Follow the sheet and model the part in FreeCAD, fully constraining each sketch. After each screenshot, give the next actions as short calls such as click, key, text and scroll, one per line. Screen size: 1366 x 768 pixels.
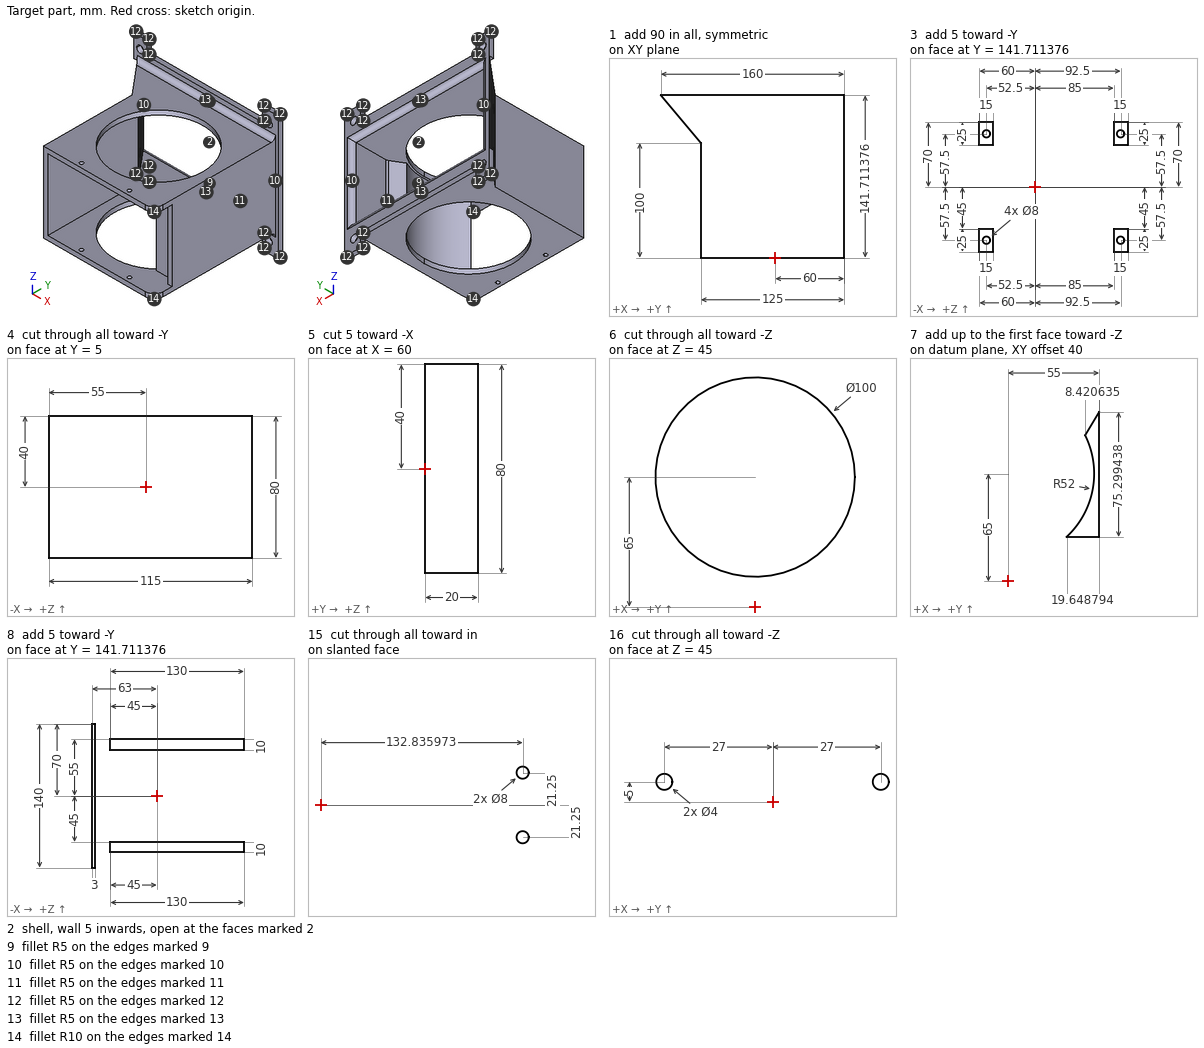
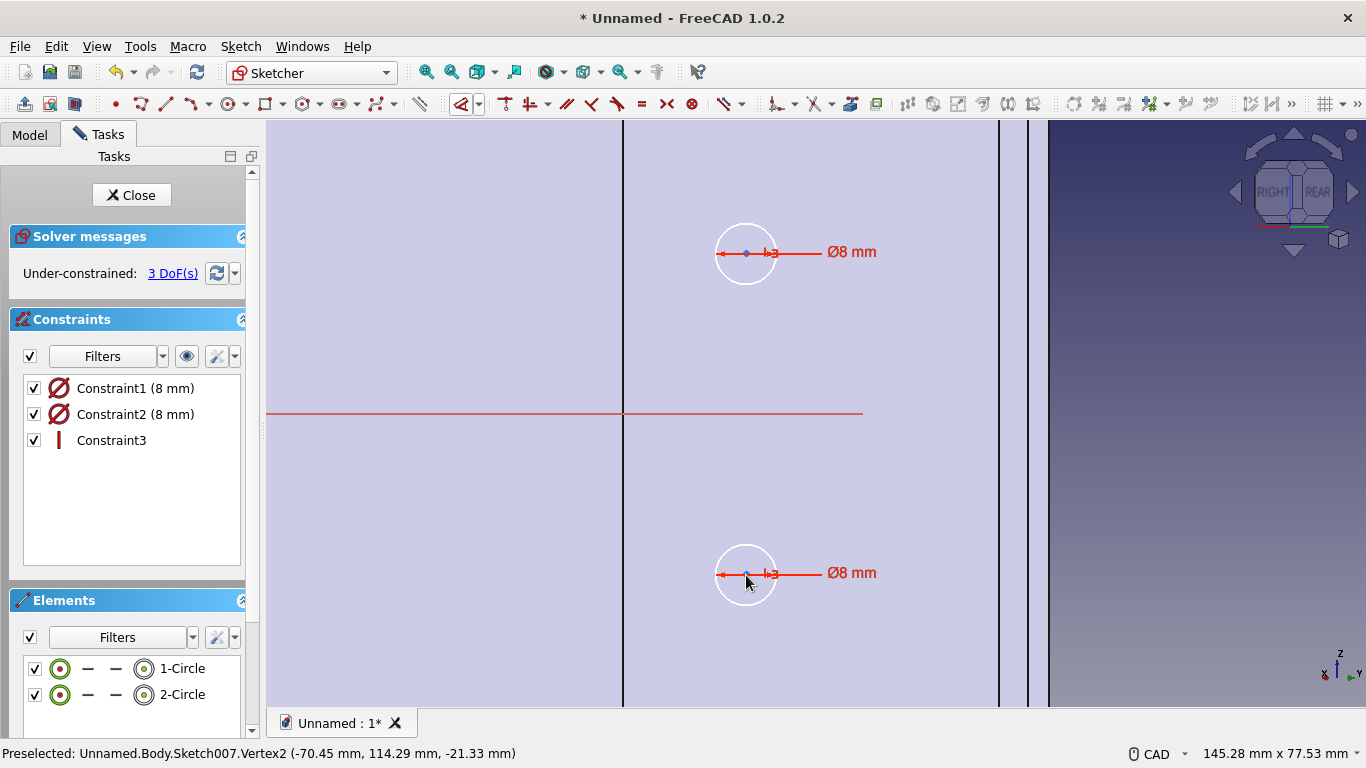
click(746, 254)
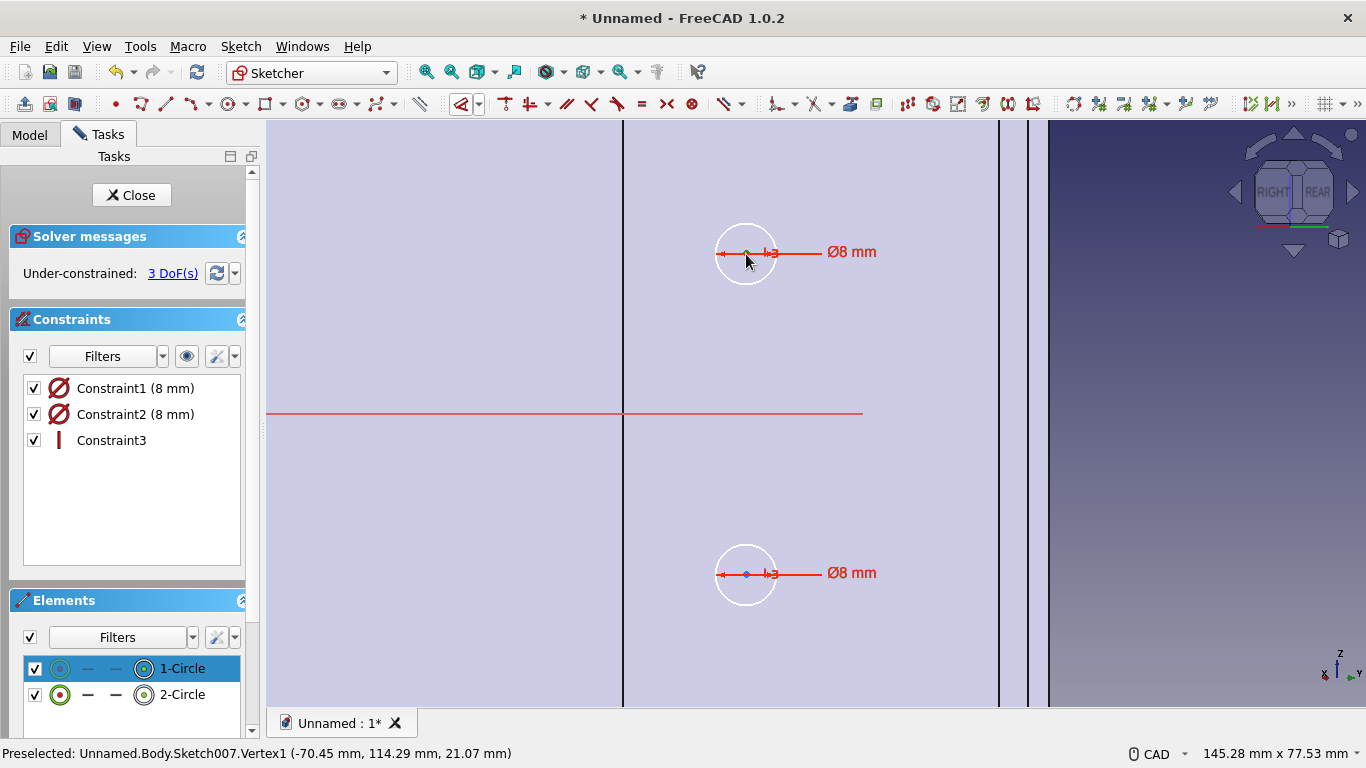
click(478, 104)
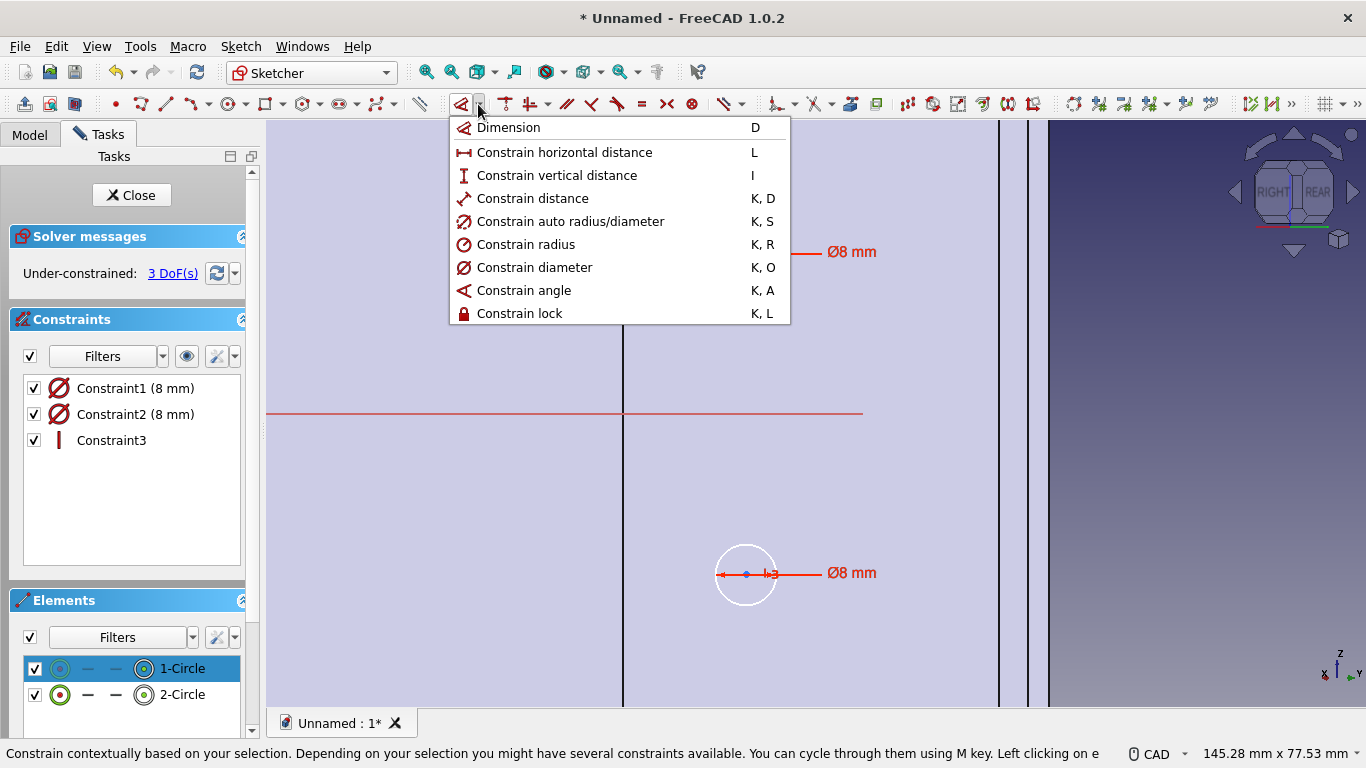
click(620, 176)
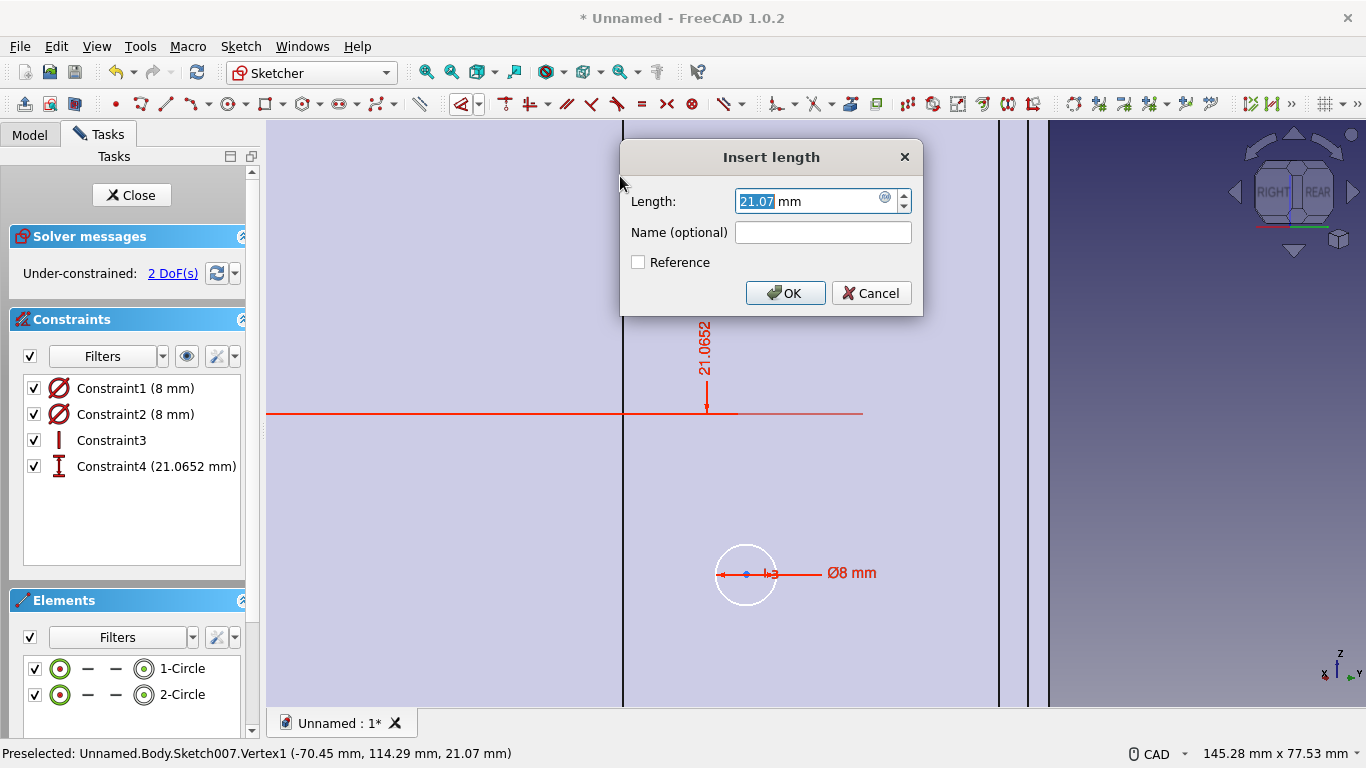
text(21.25)
key(Return)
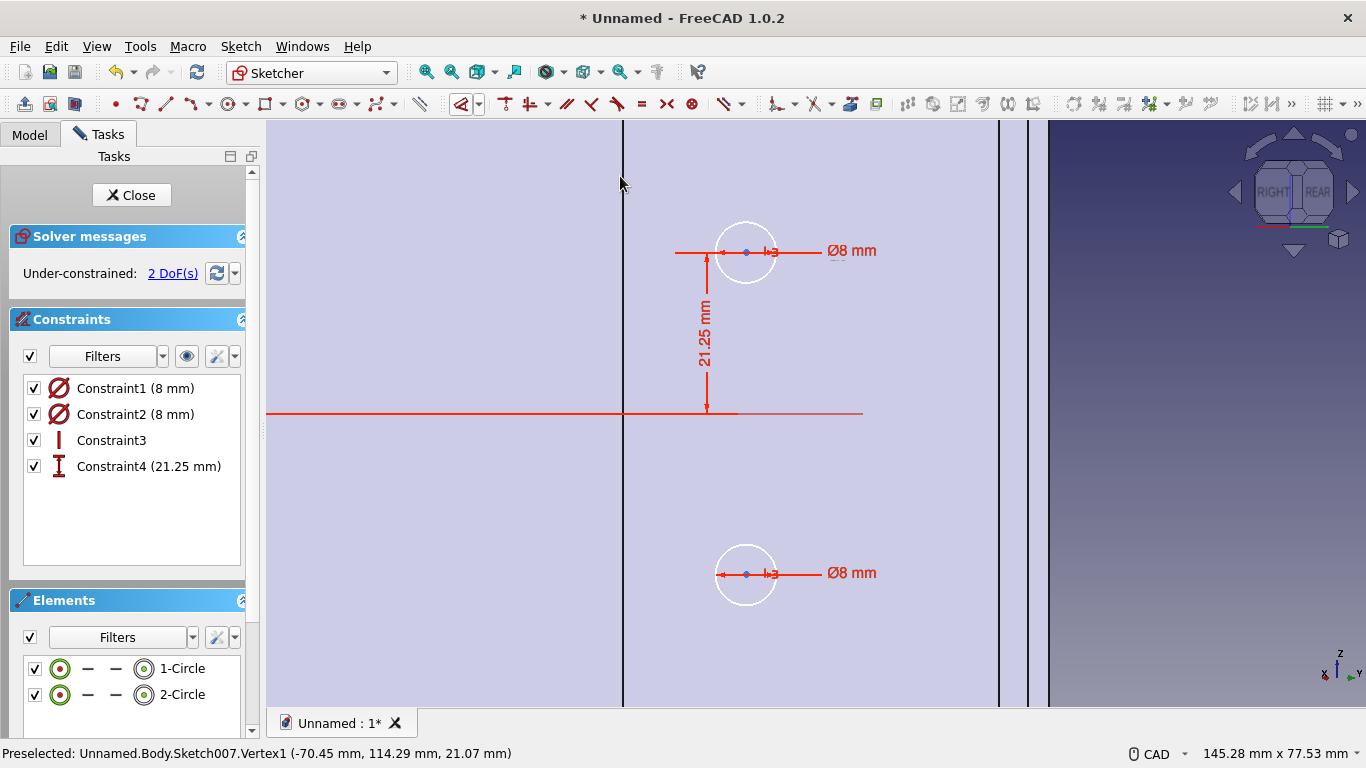
click(746, 575)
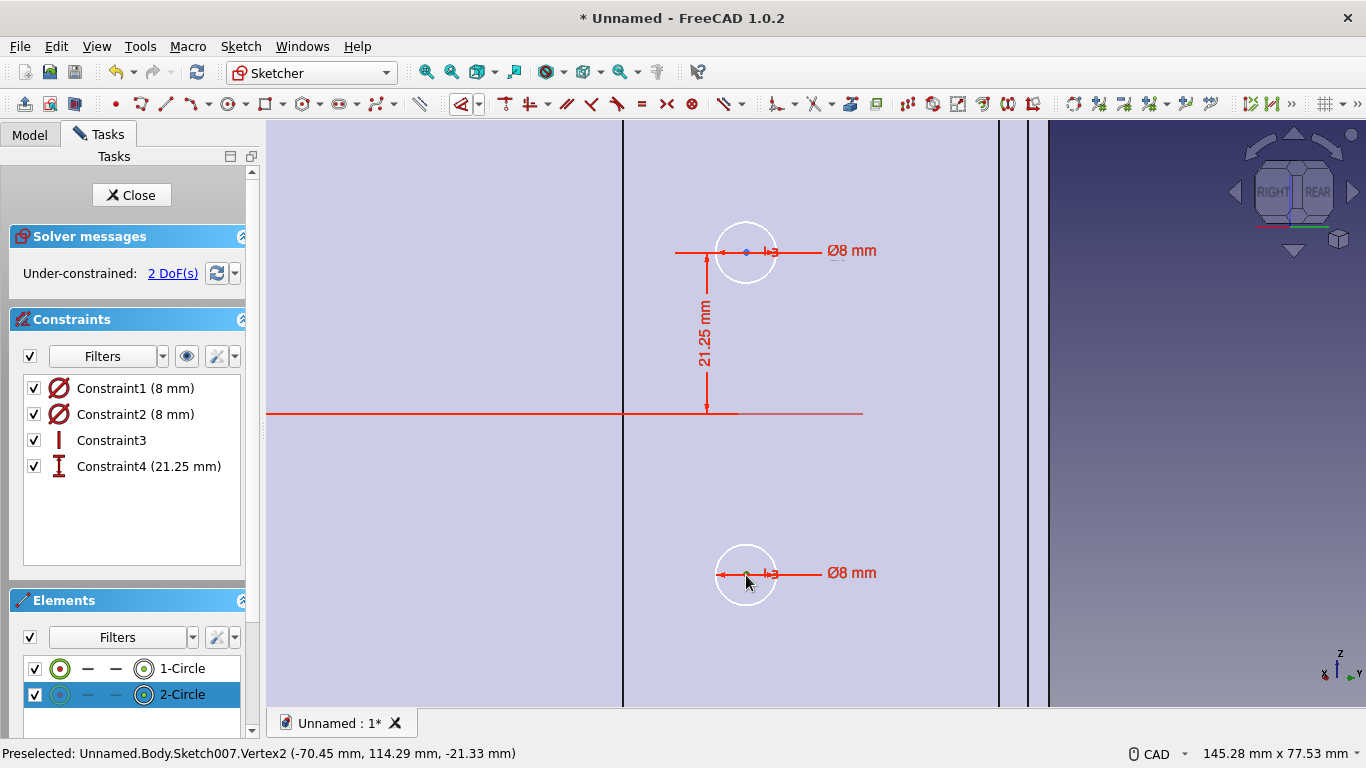
key(i)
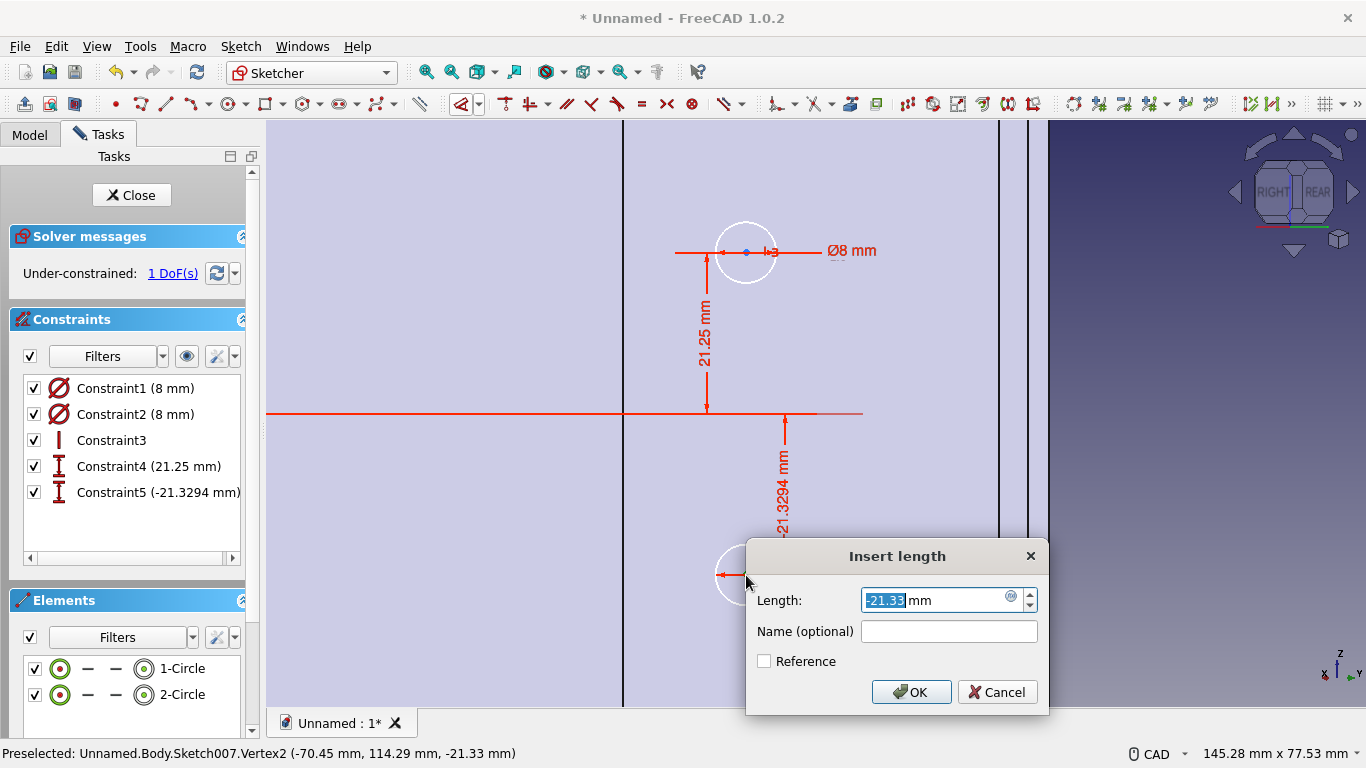
text(-21.25)
key(Return)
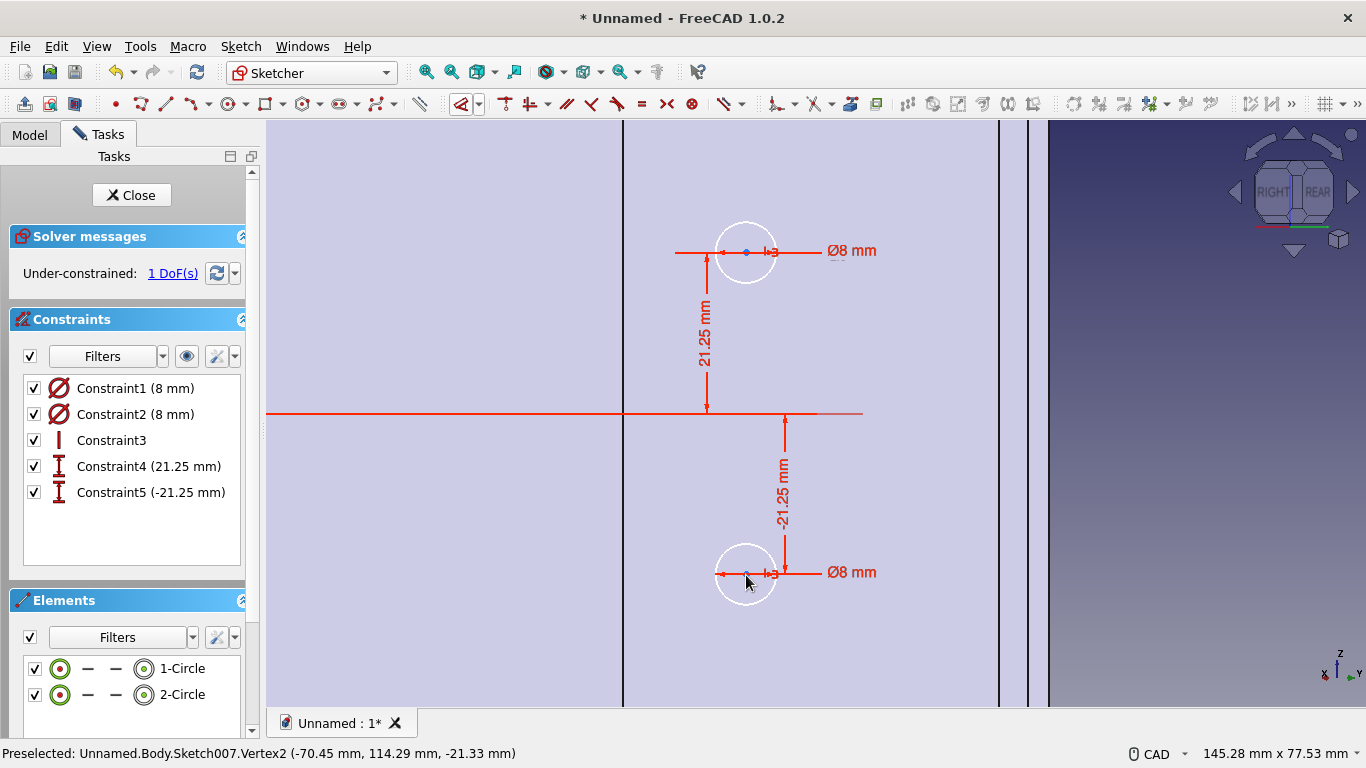
click(746, 253)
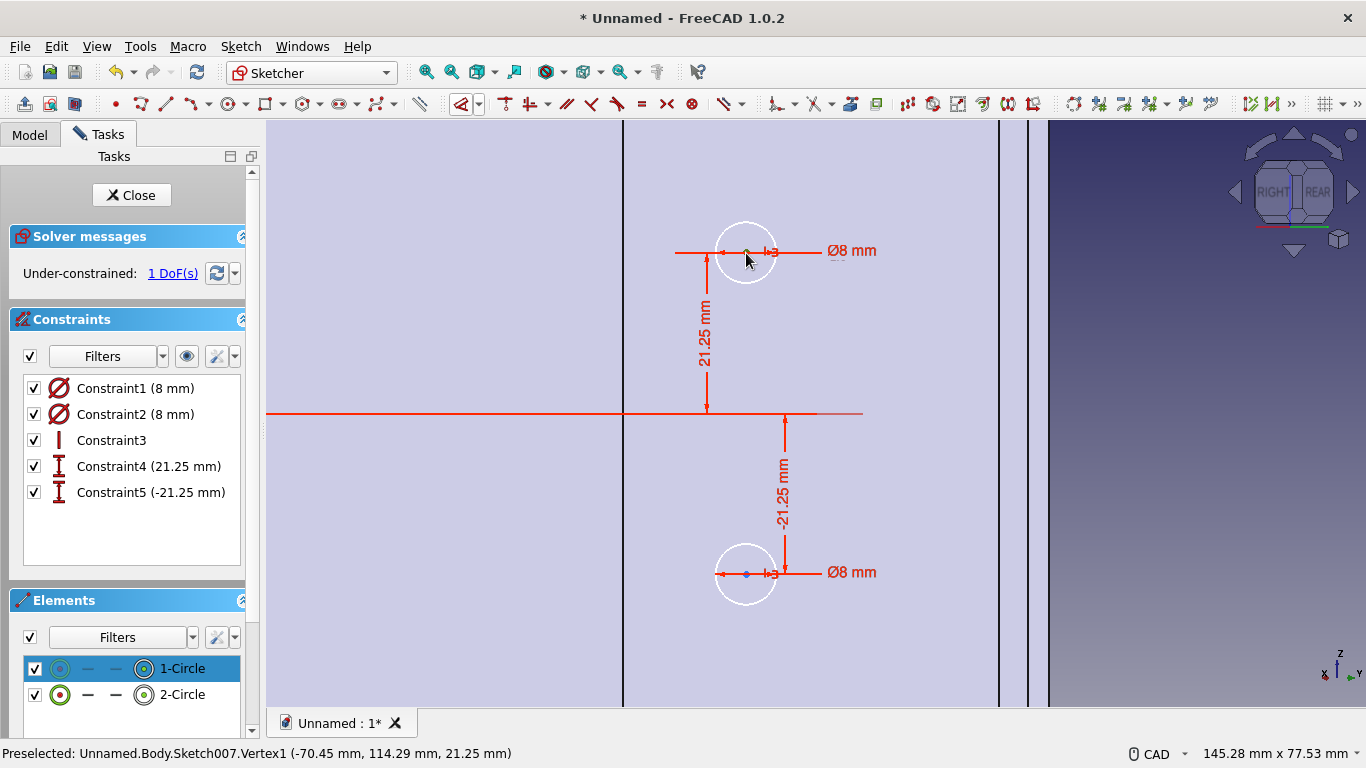
key(l)